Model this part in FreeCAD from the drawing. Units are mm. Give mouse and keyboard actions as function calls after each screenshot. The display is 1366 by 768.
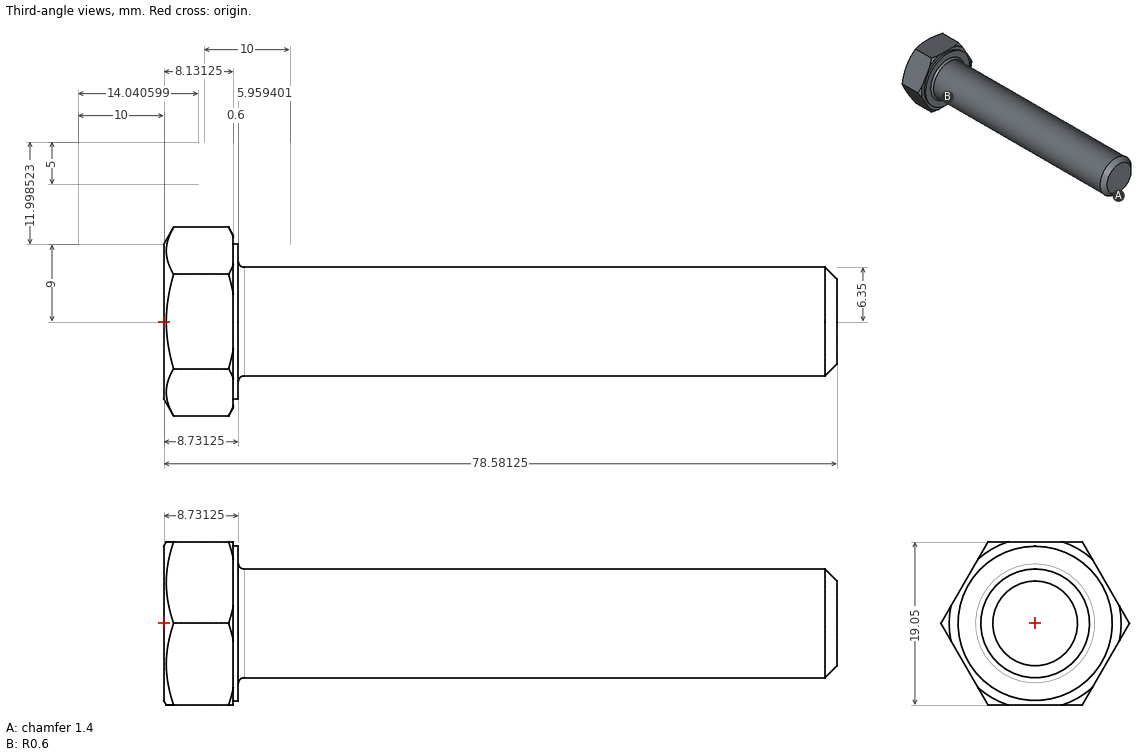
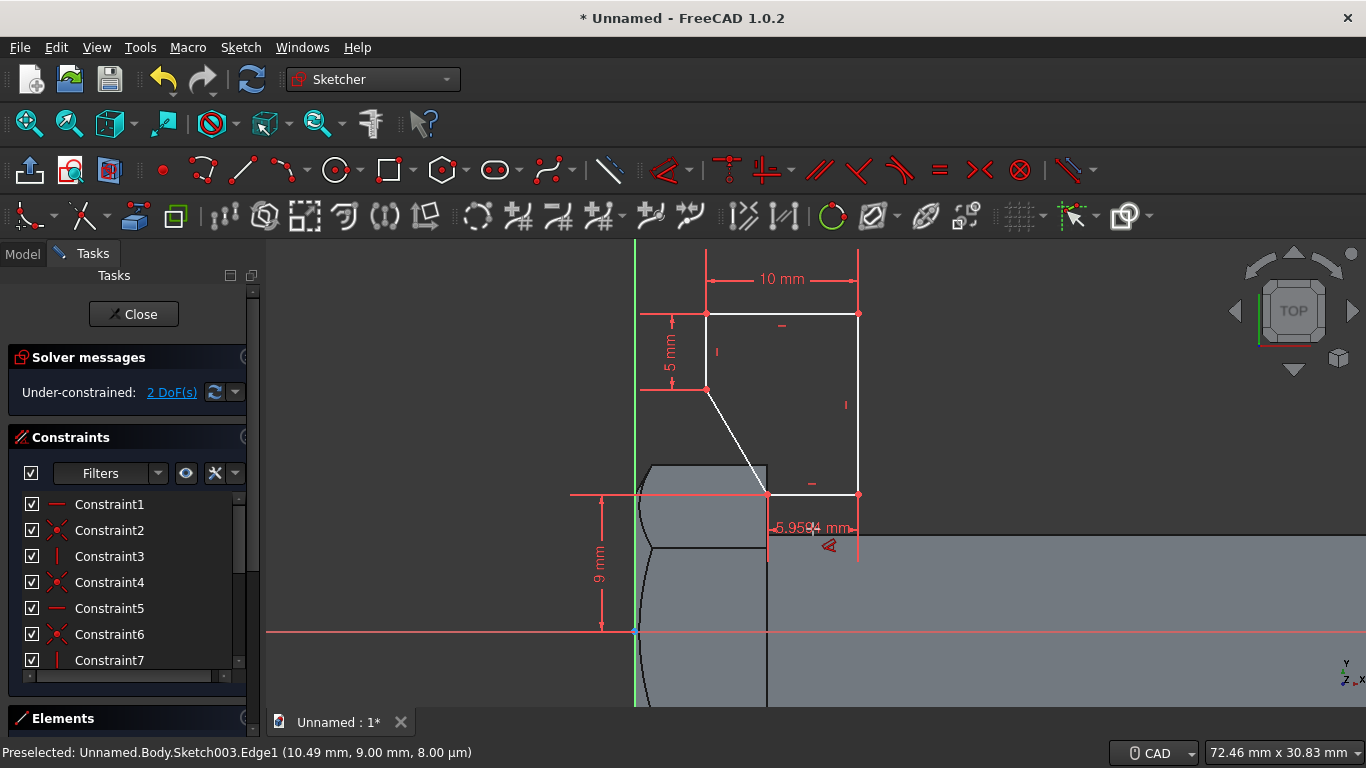
click(768, 495)
click(701, 665)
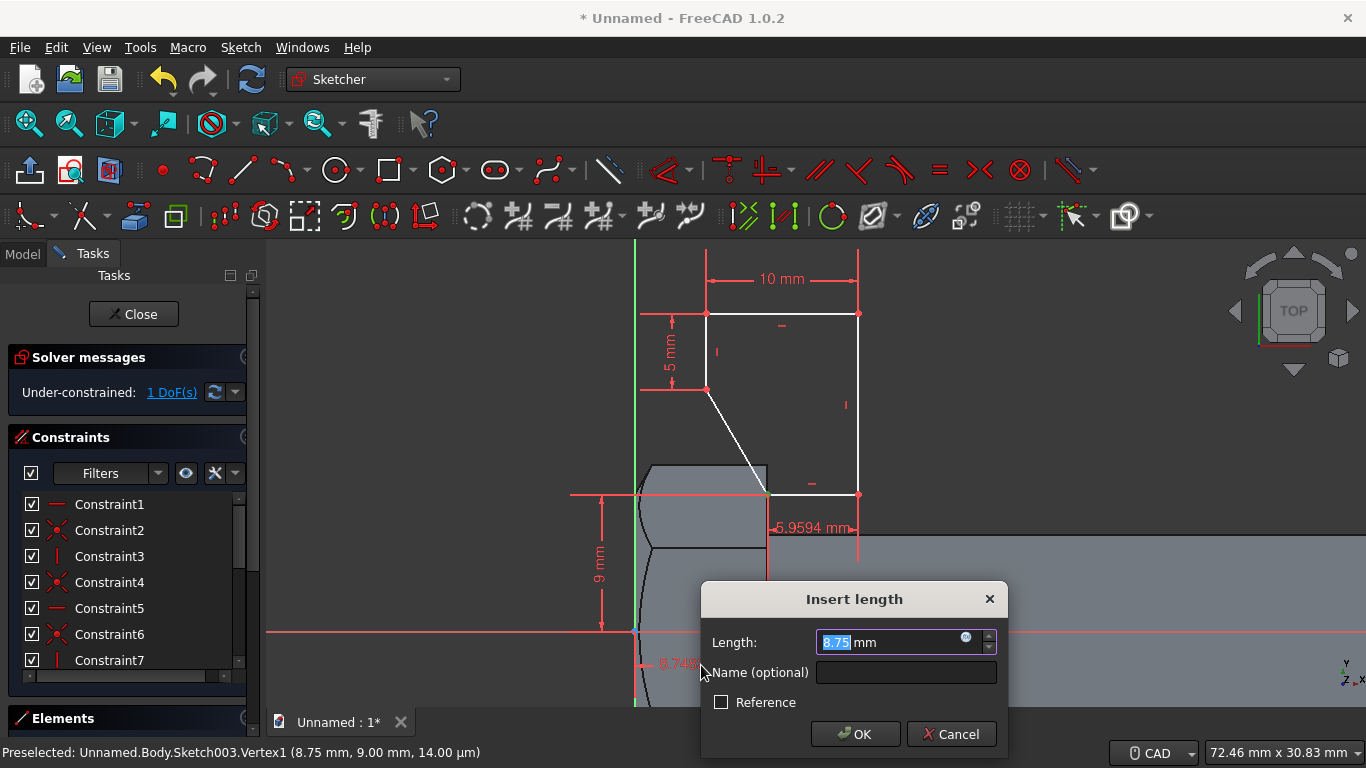
text(8.73125)
key(Return)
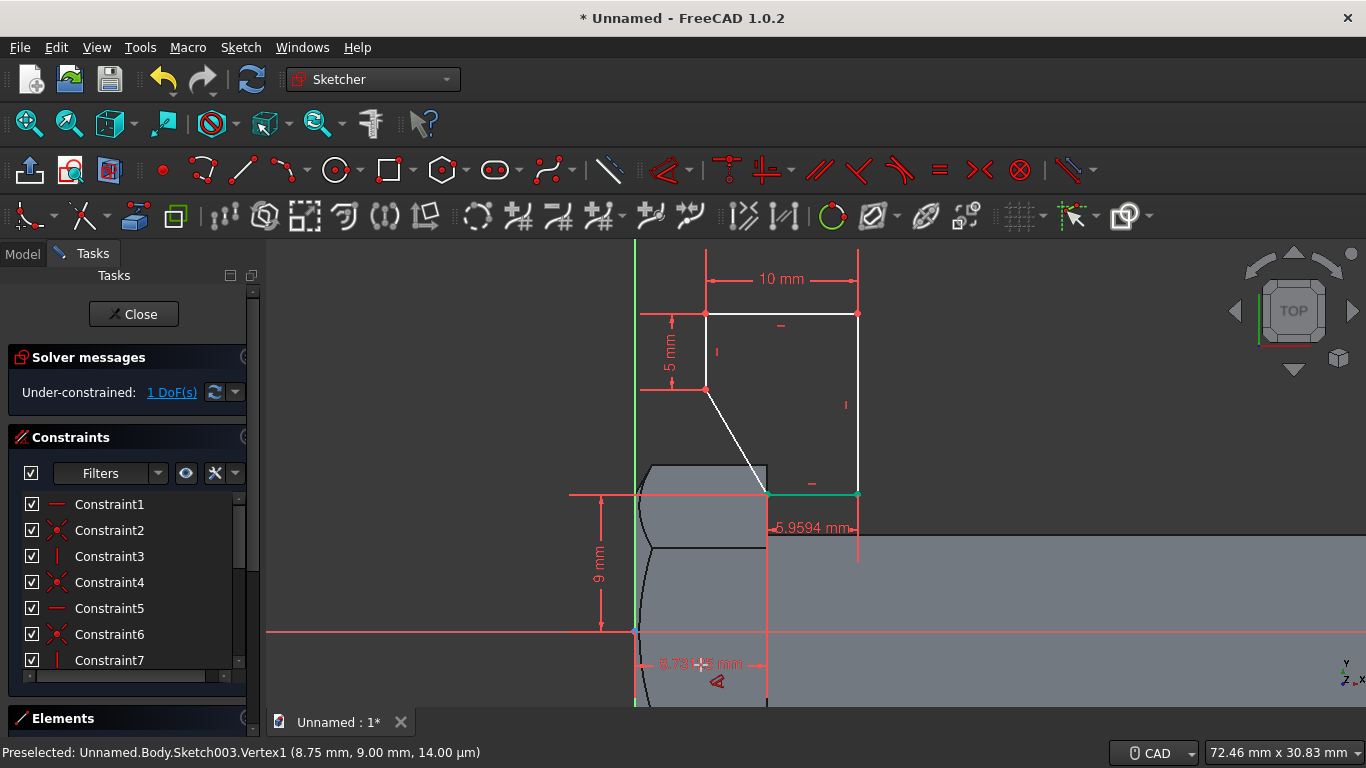
click(858, 441)
click(892, 404)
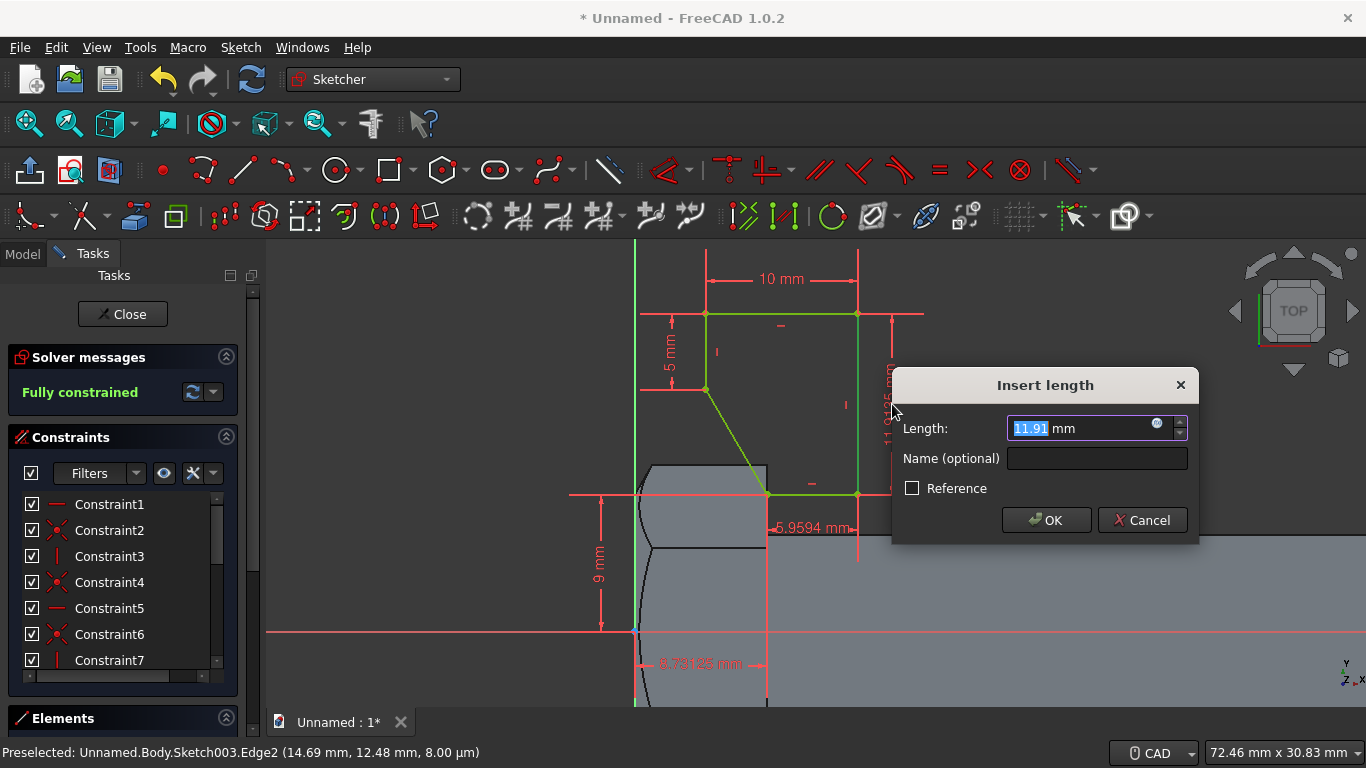
text(11.998523)
key(Return)
key(Escape)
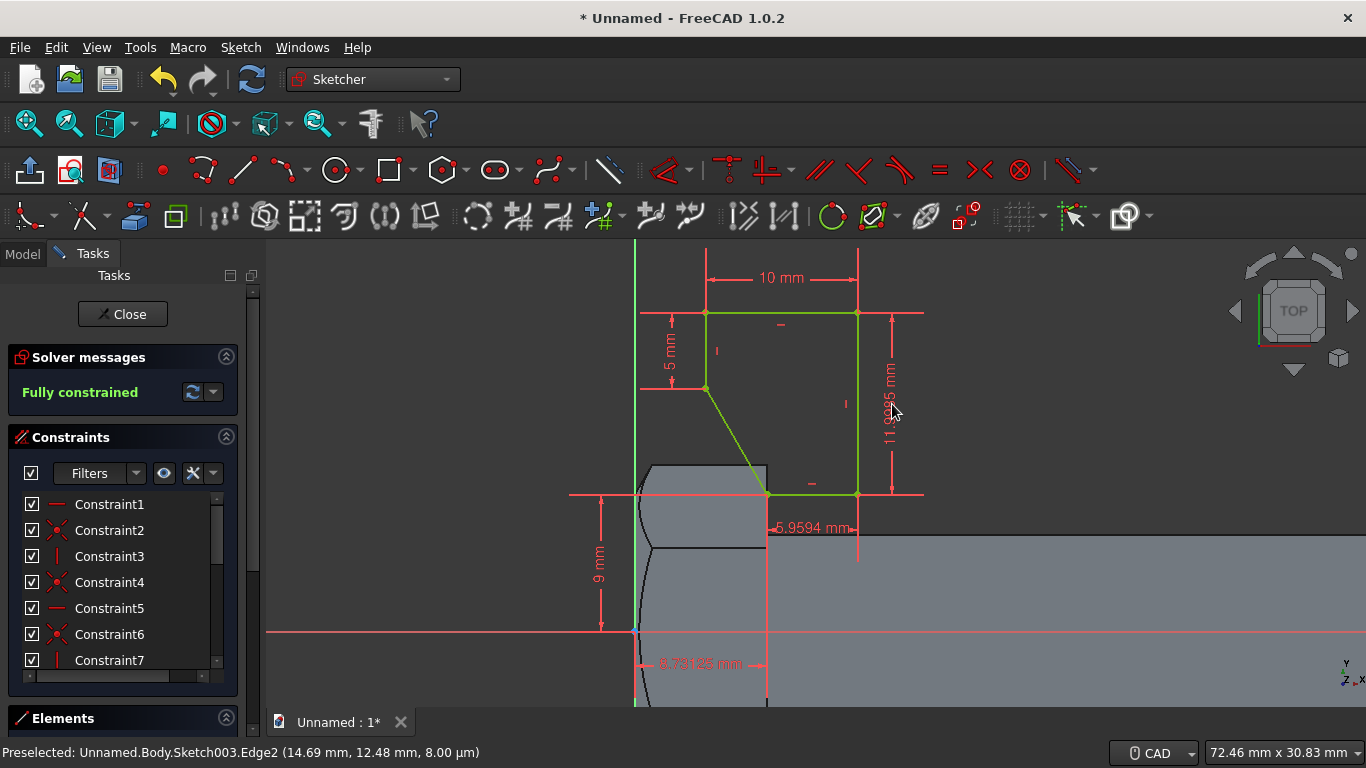
click(123, 314)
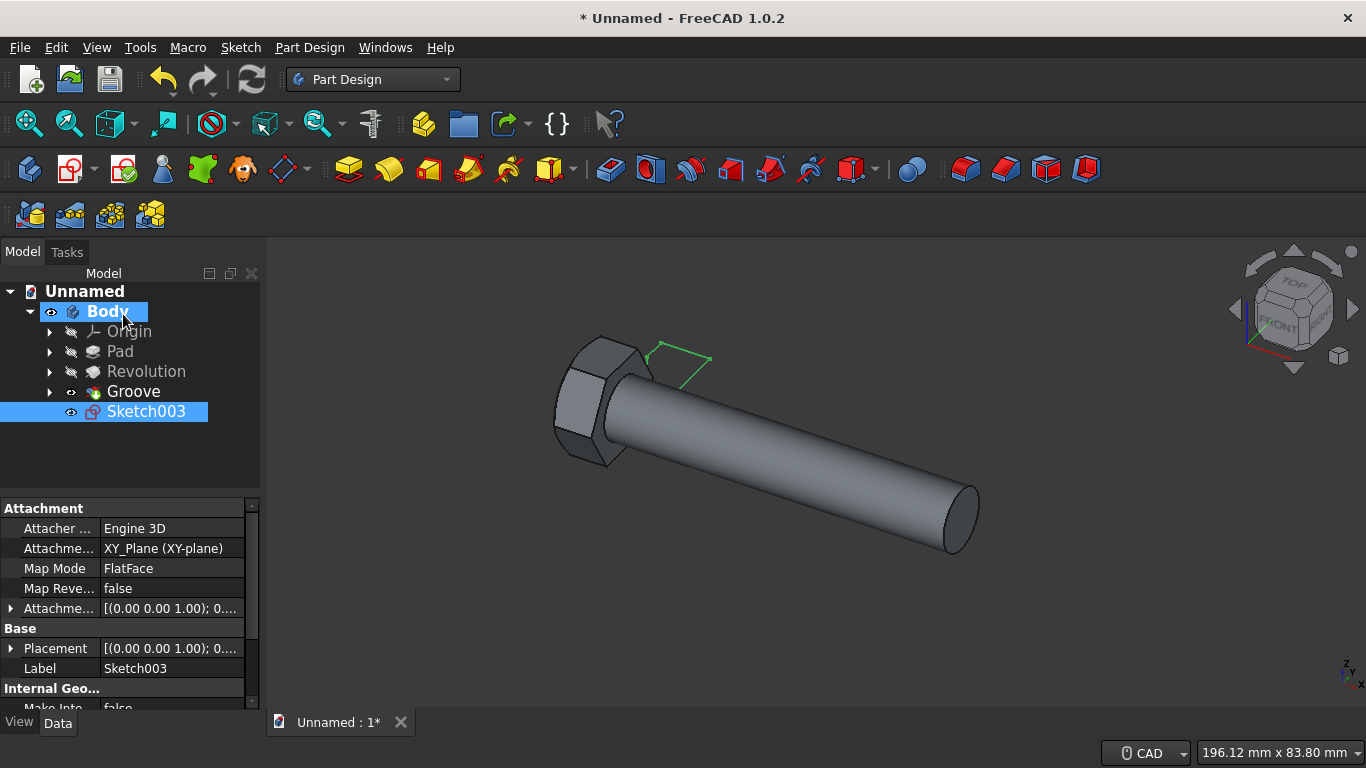
click(692, 170)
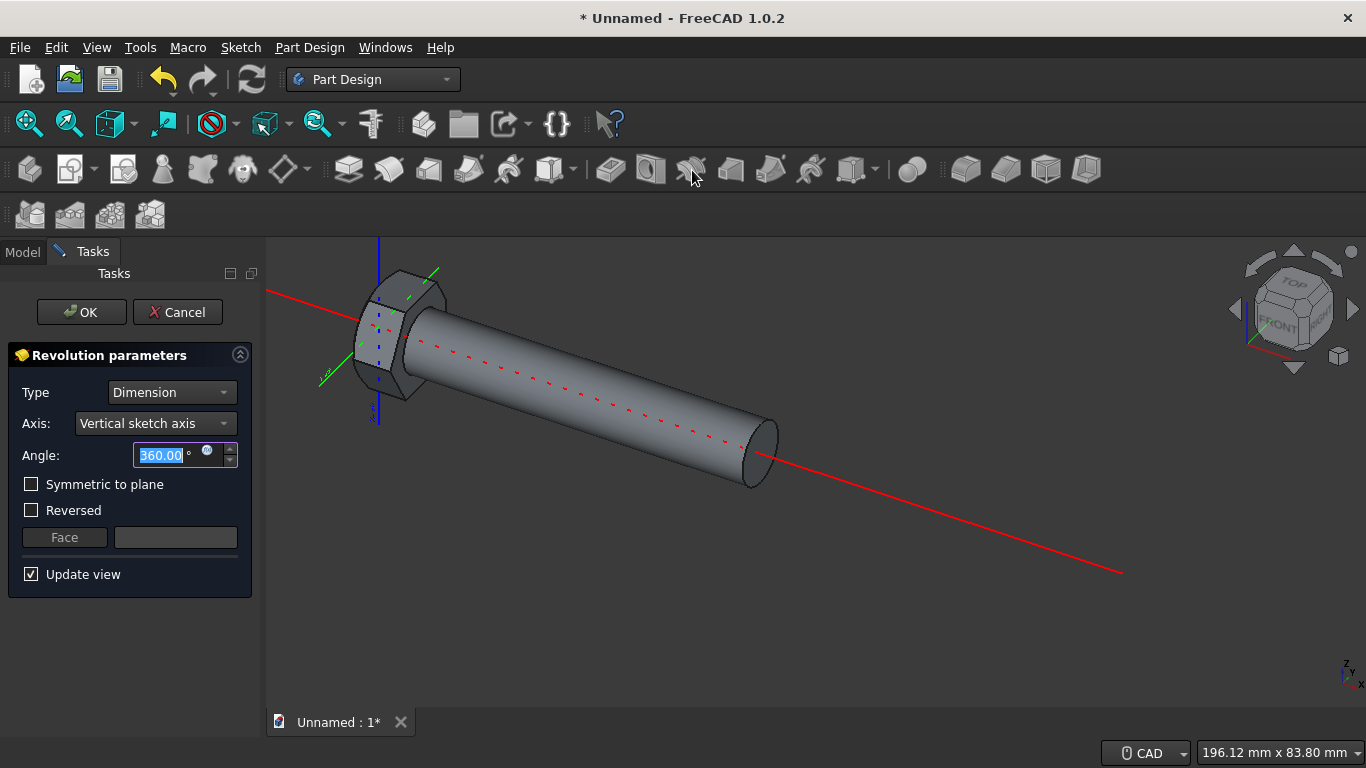
click(156, 424)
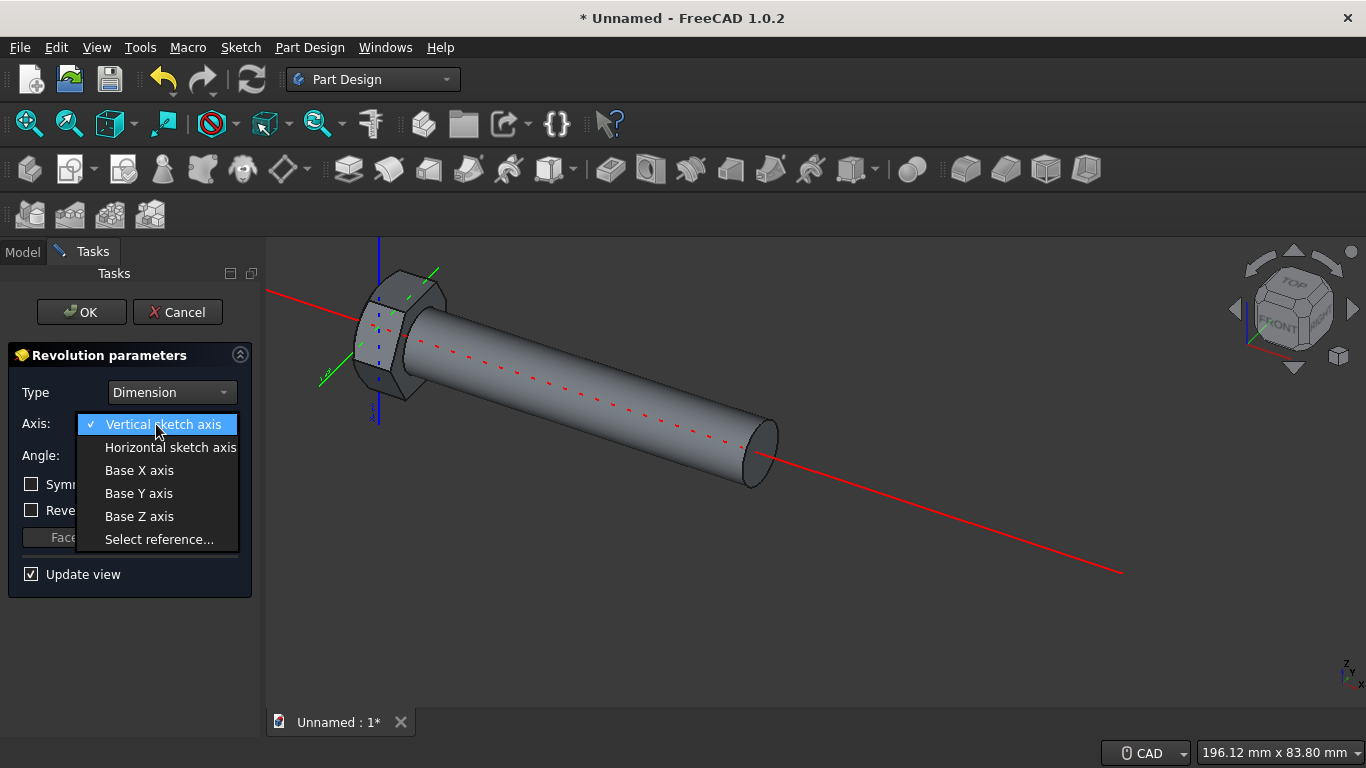
click(156, 448)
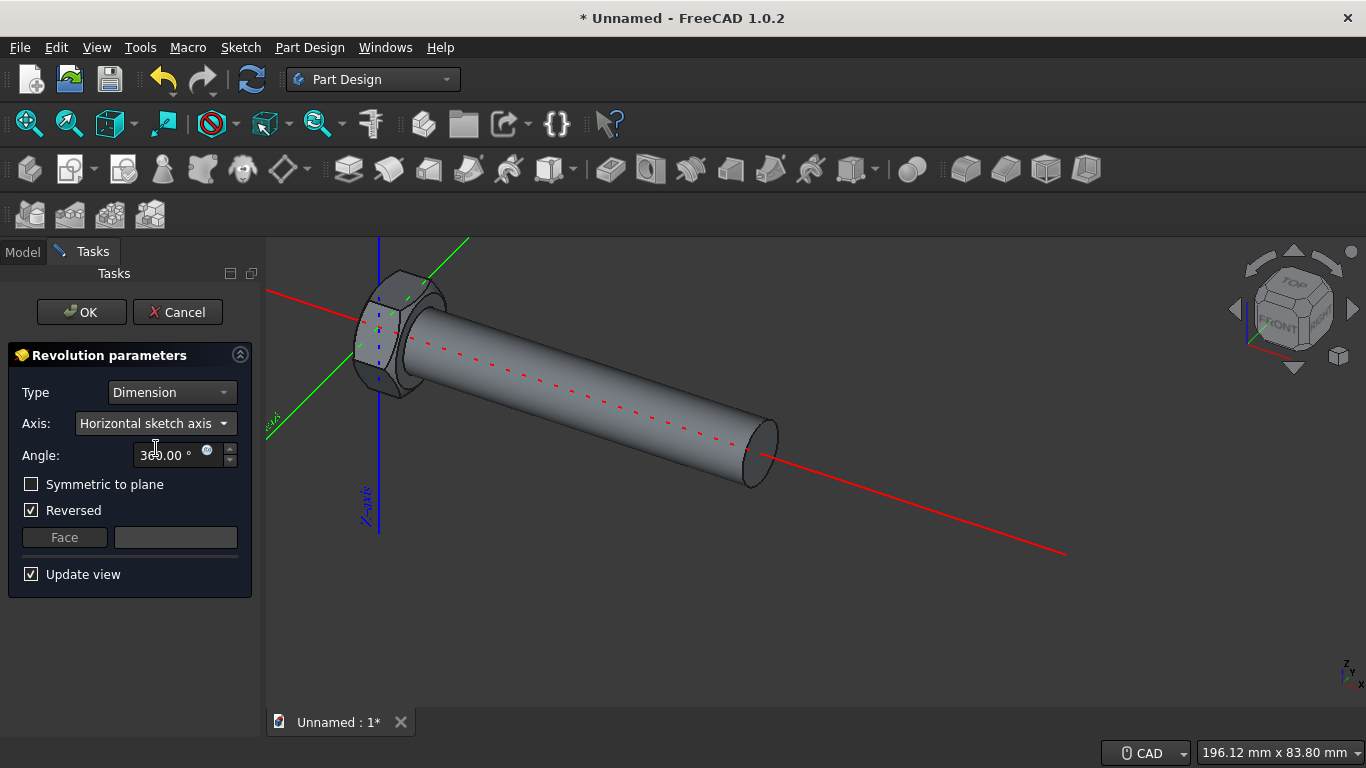
click(82, 312)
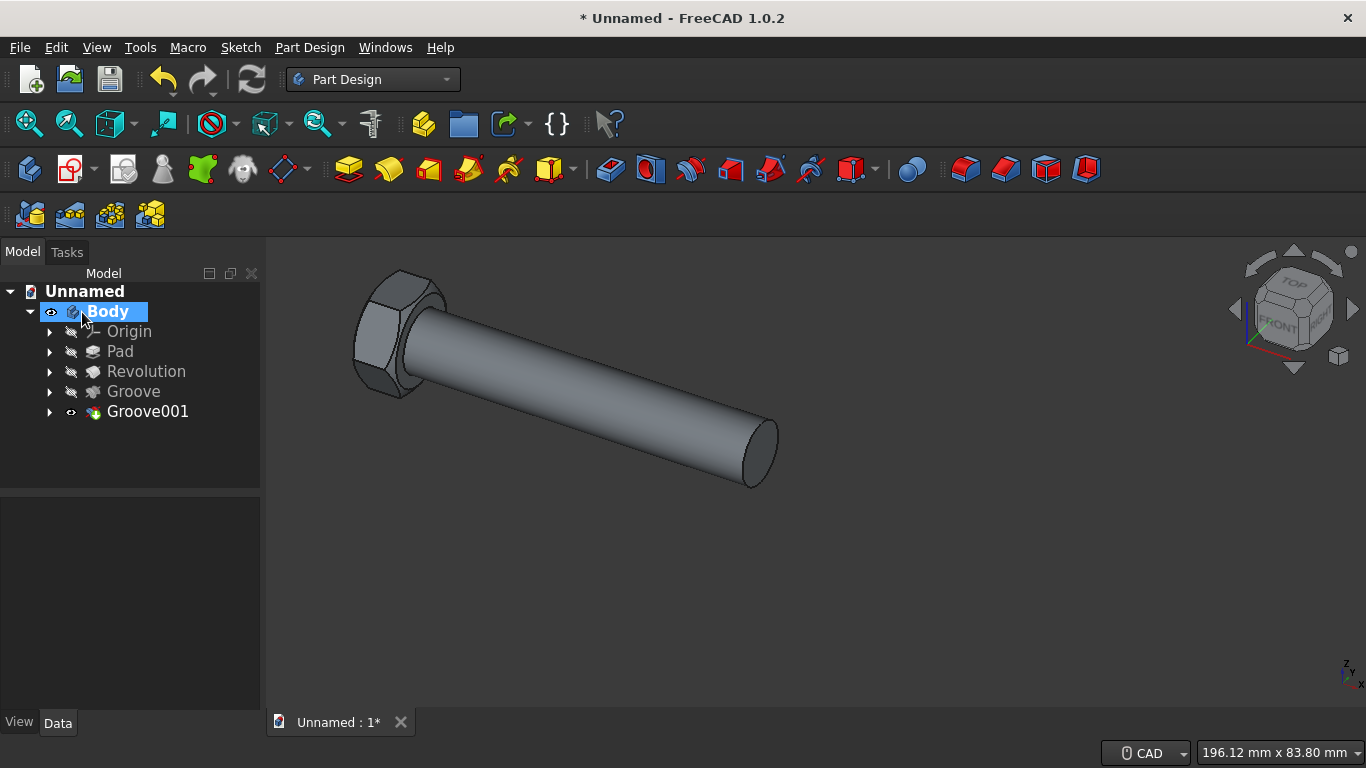
click(70, 170)